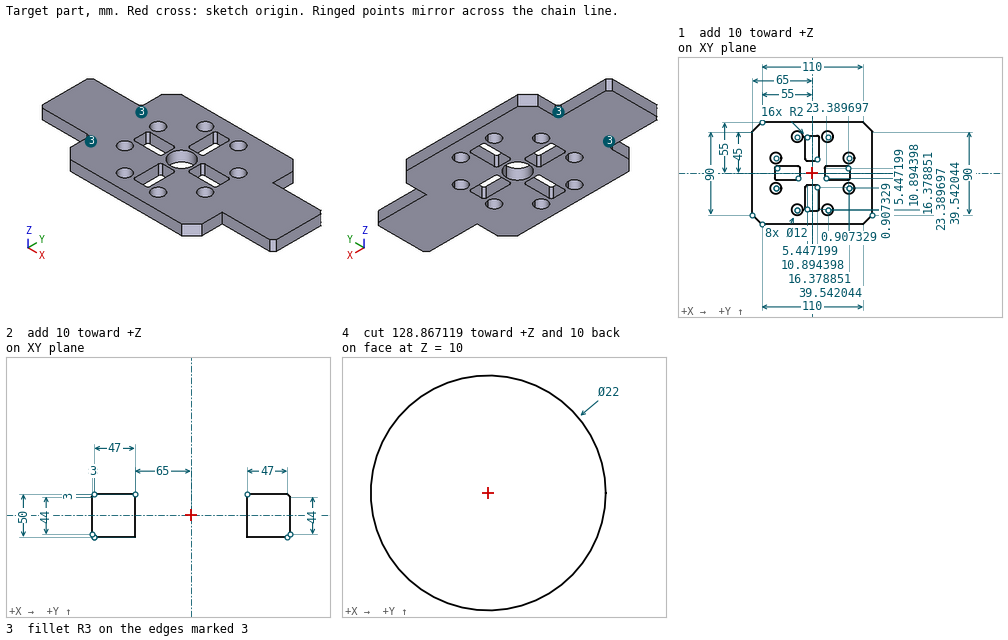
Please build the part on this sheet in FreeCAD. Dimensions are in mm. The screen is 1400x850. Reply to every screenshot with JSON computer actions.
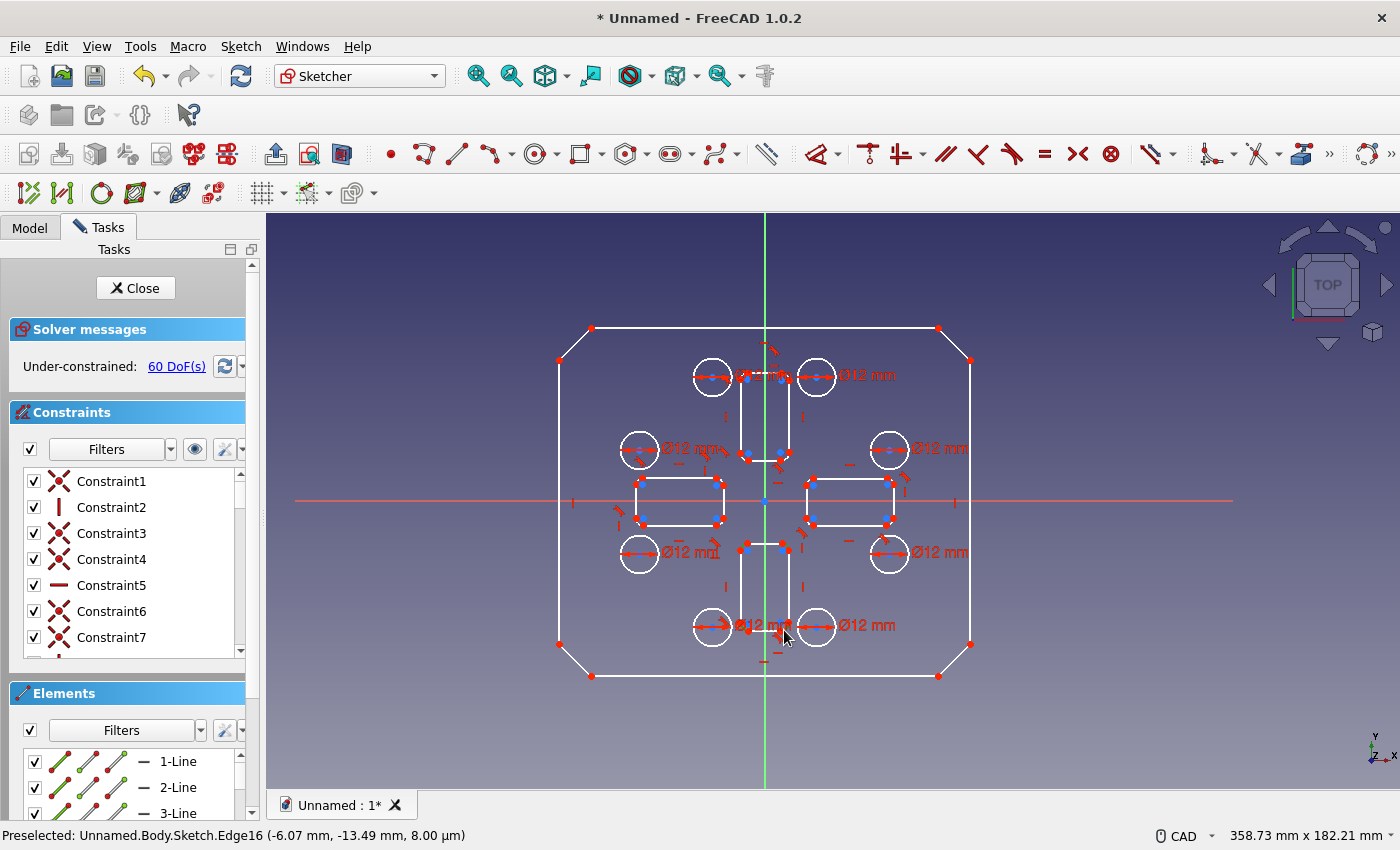
{"action": "scroll", "coordinate": [810, 479], "scroll_direction": "up", "scroll_amount": 8}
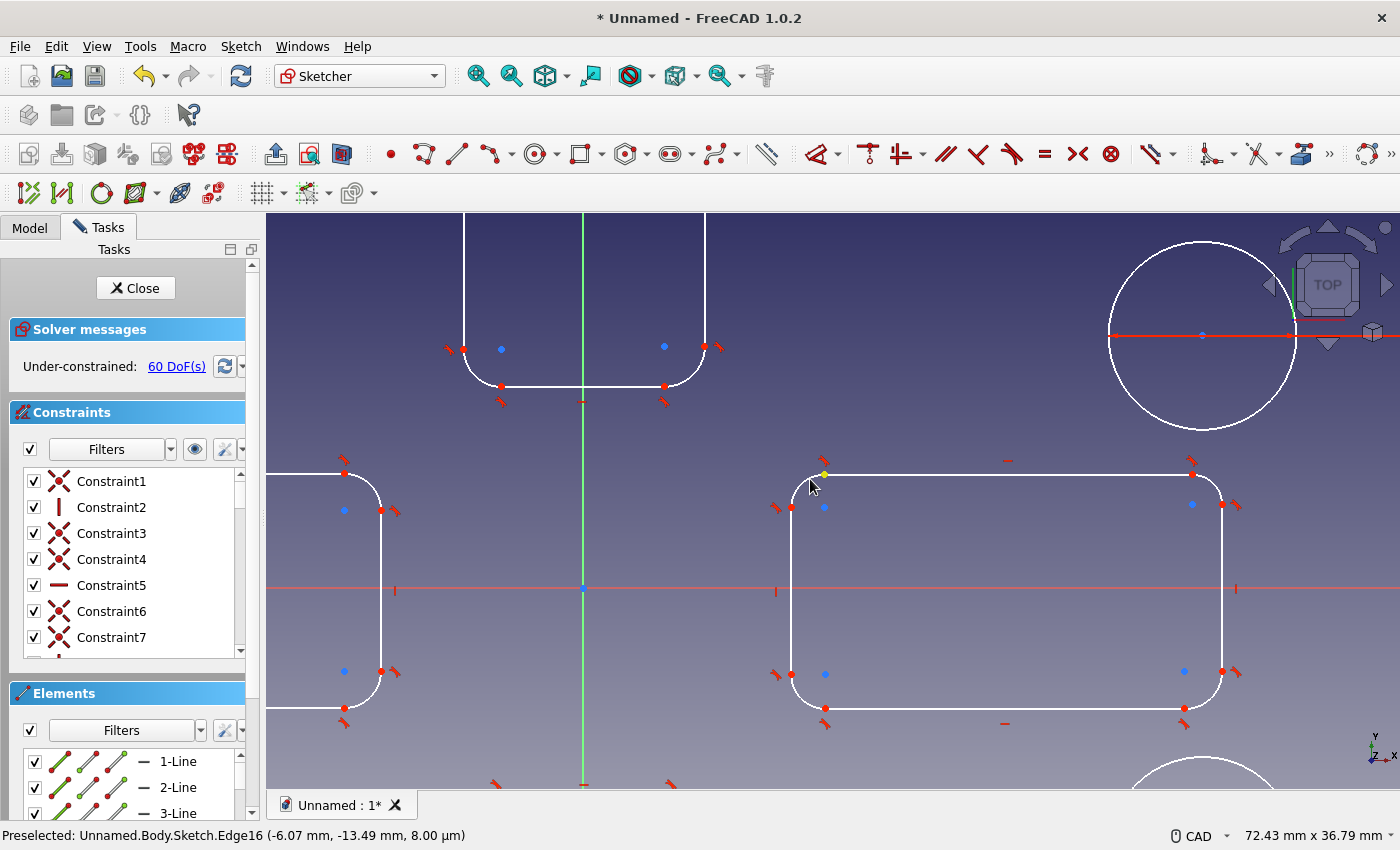
{"action": "left_click", "coordinate": [809, 478]}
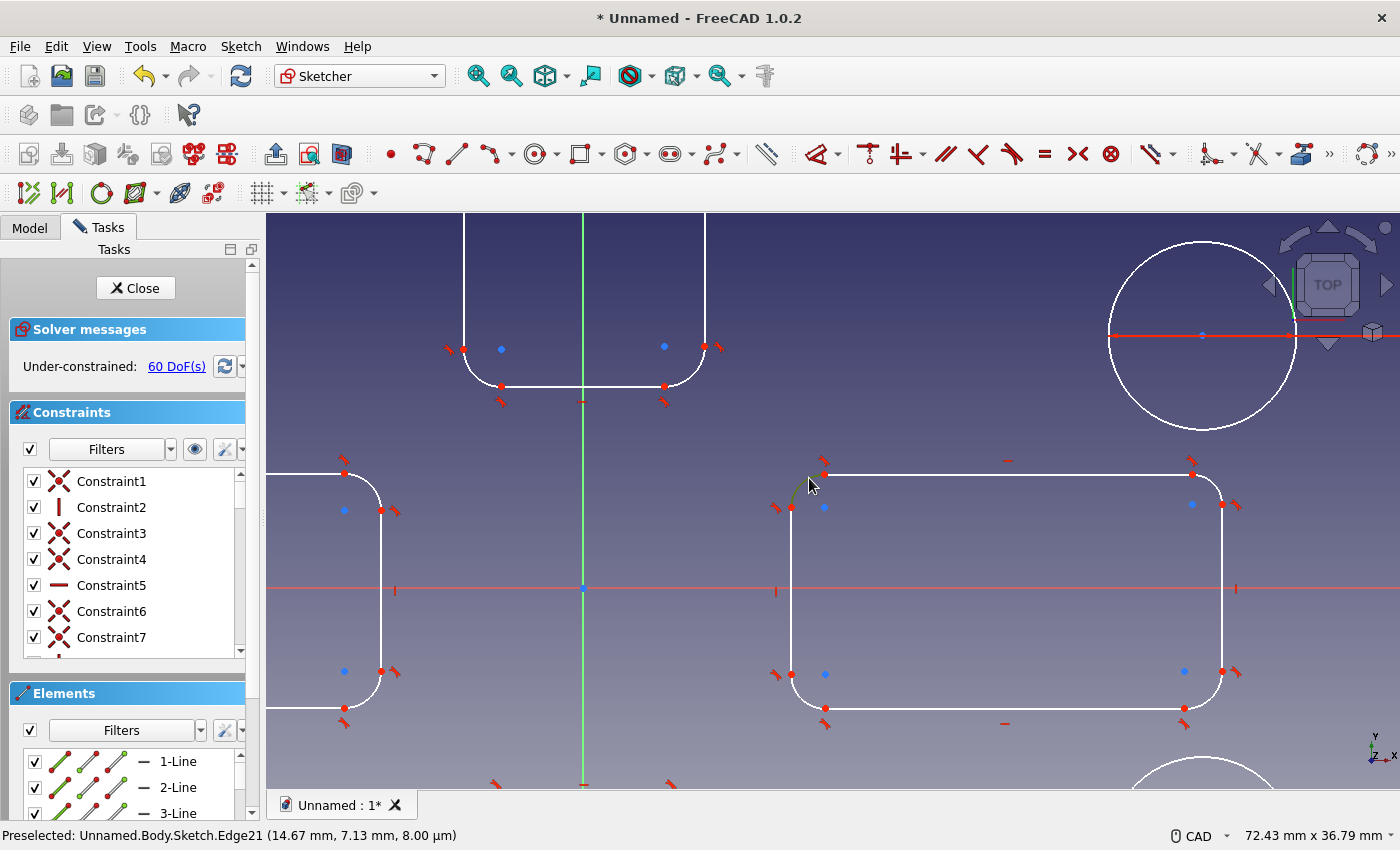
{"action": "left_click", "coordinate": [1219, 491]}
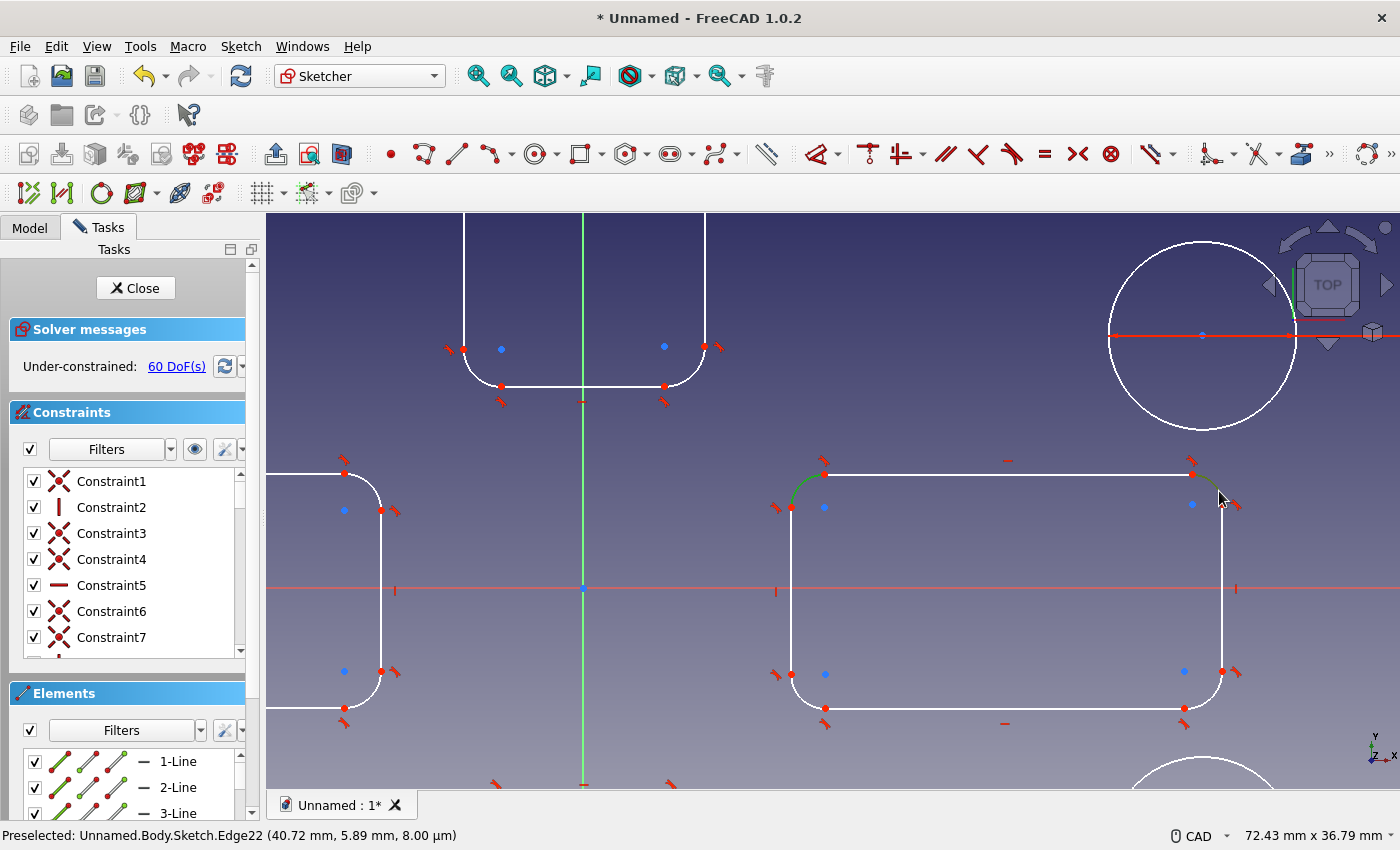
{"action": "left_click", "coordinate": [1202, 705]}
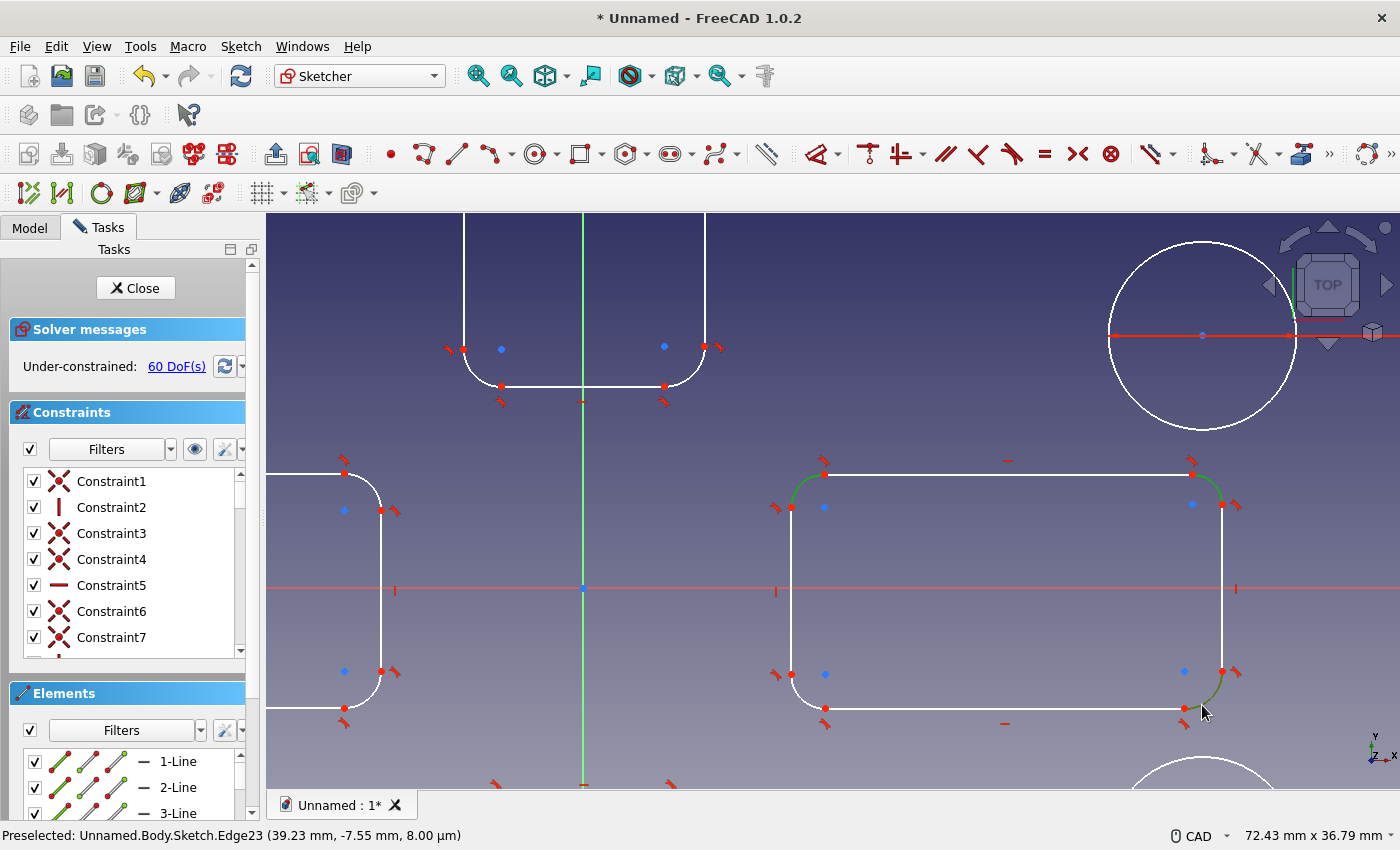
{"action": "left_click", "coordinate": [795, 690]}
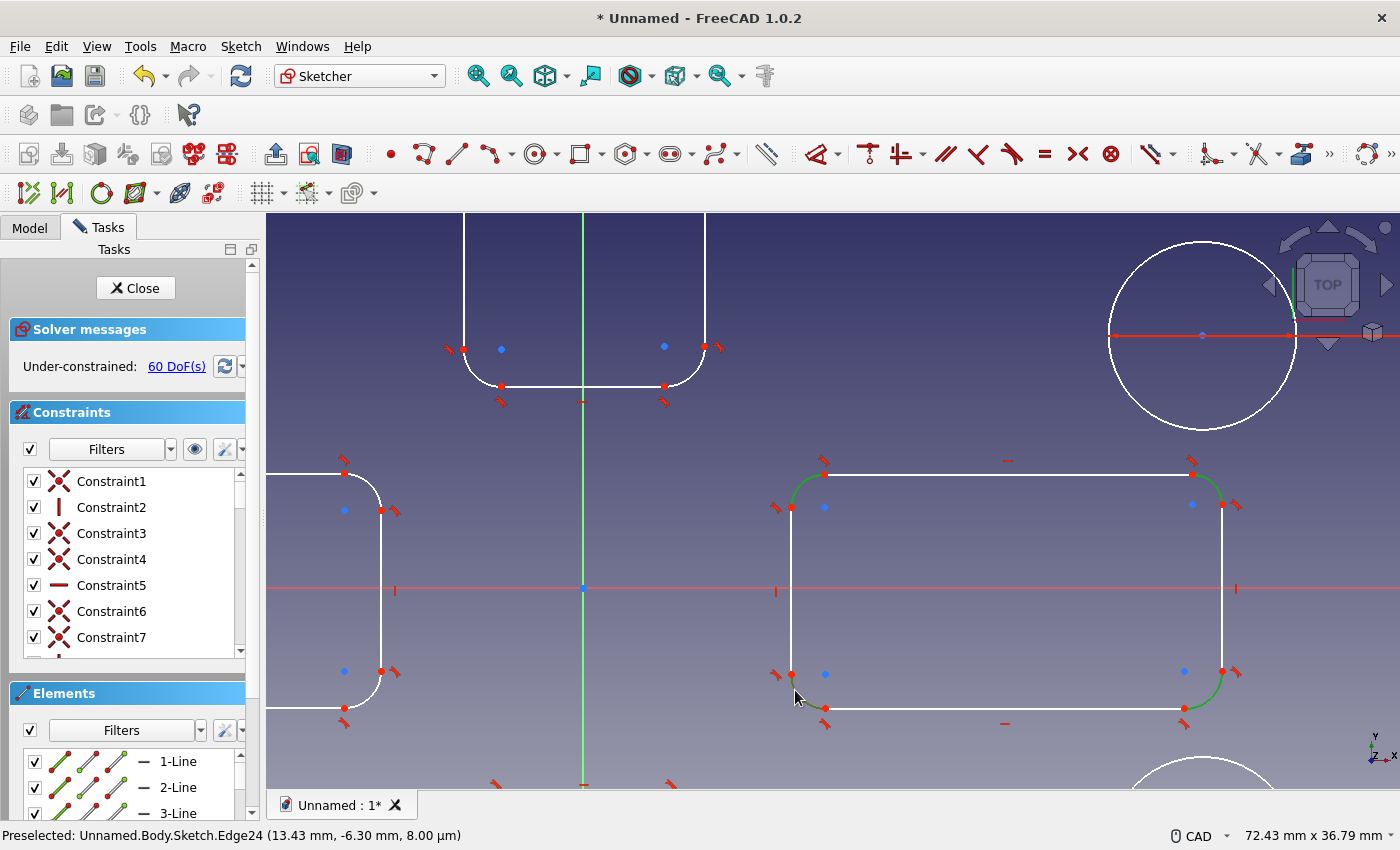
{"action": "left_click", "coordinate": [361, 704]}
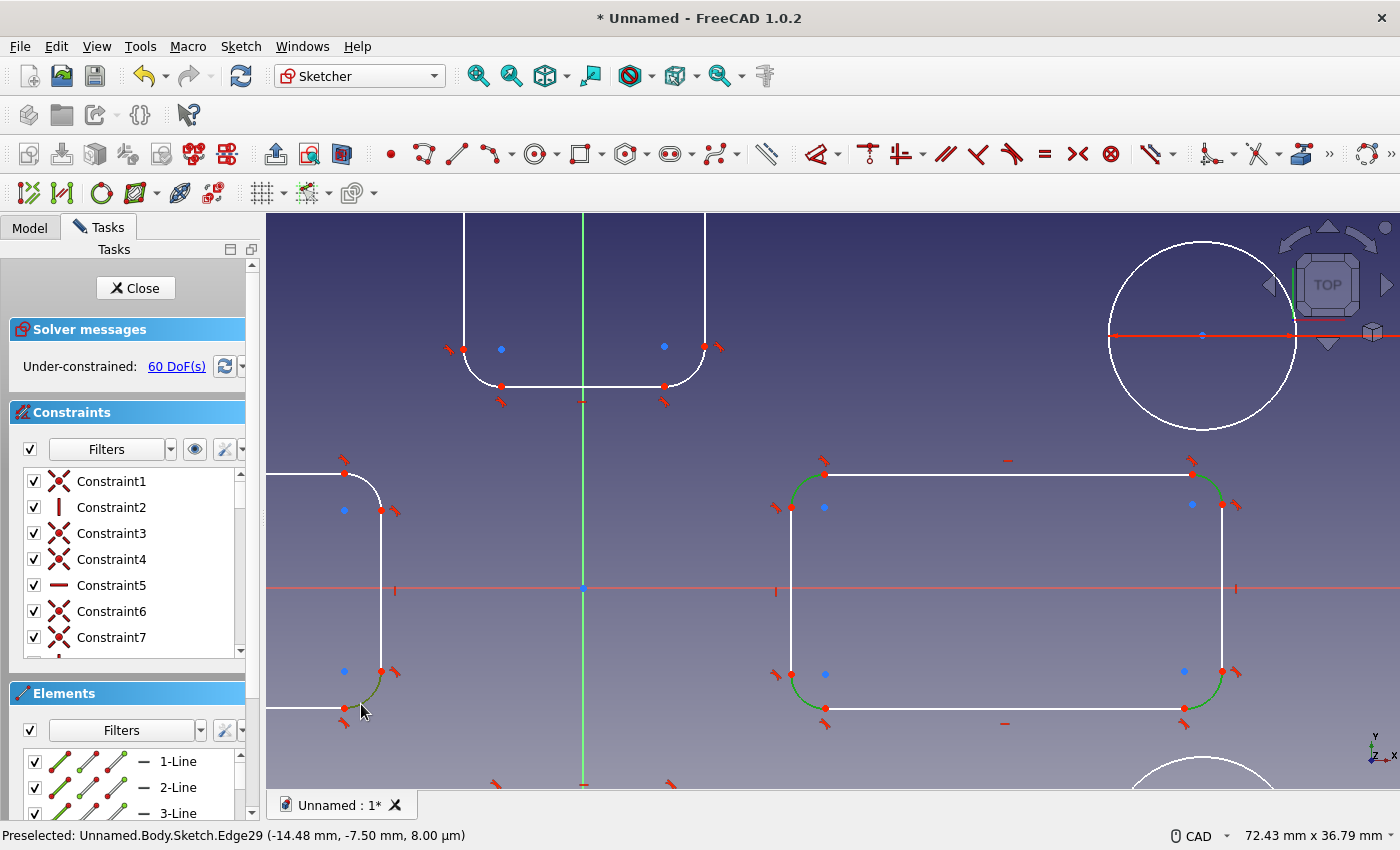
{"action": "scroll", "coordinate": [810, 479], "scroll_direction": "down", "scroll_amount": 8}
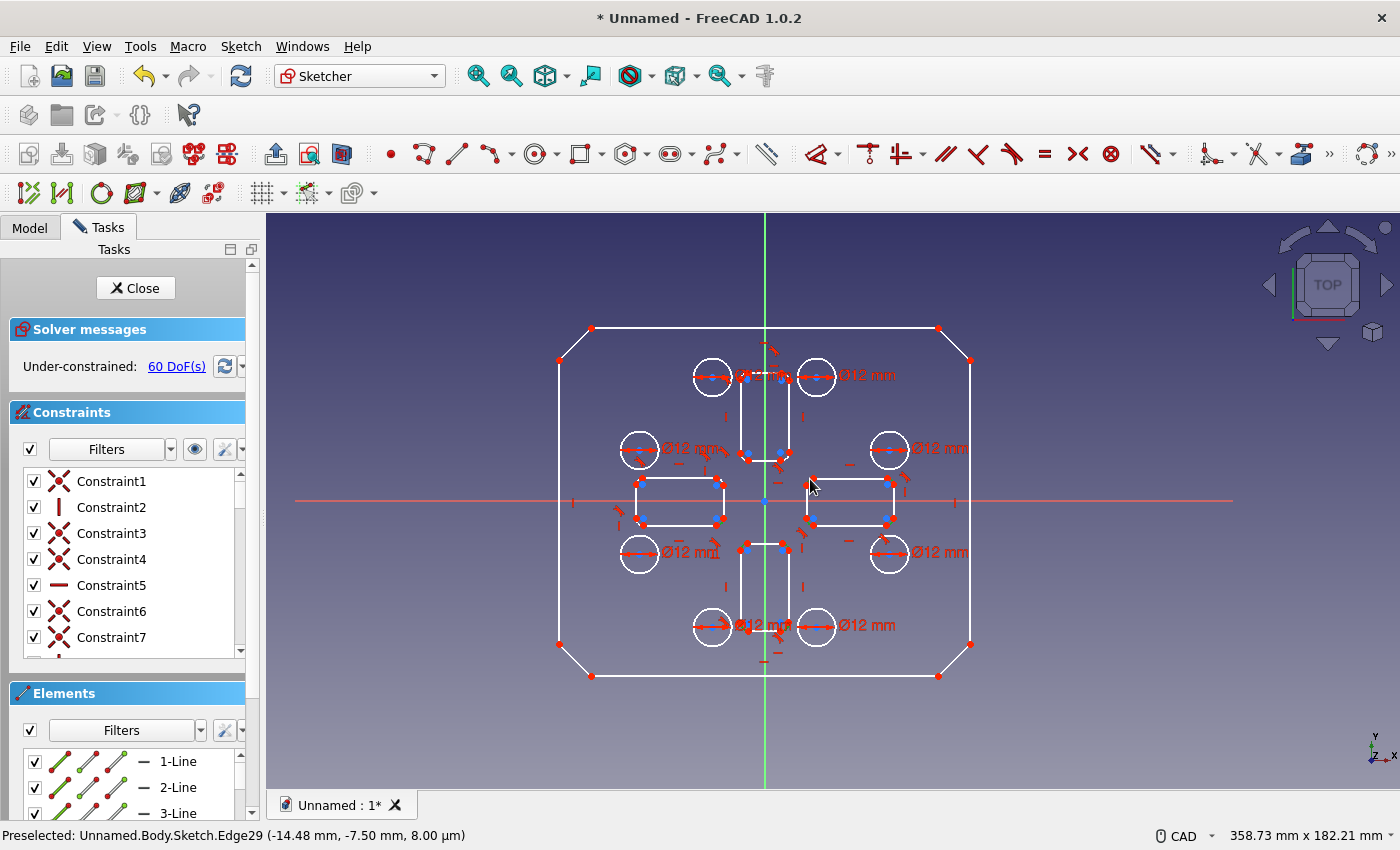
{"action": "scroll", "coordinate": [637, 522], "scroll_direction": "up", "scroll_amount": 8}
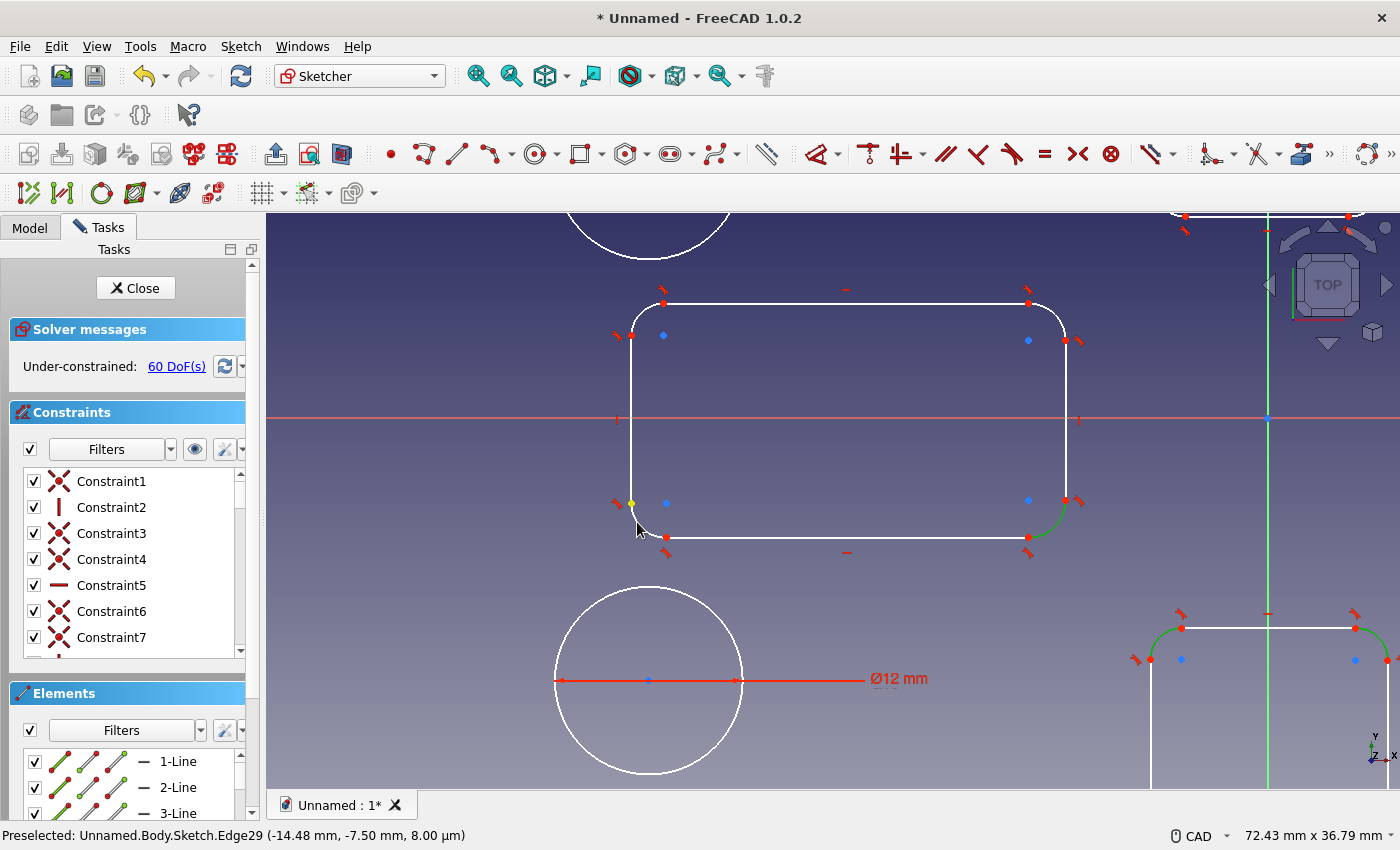
{"action": "left_click", "coordinate": [635, 519]}